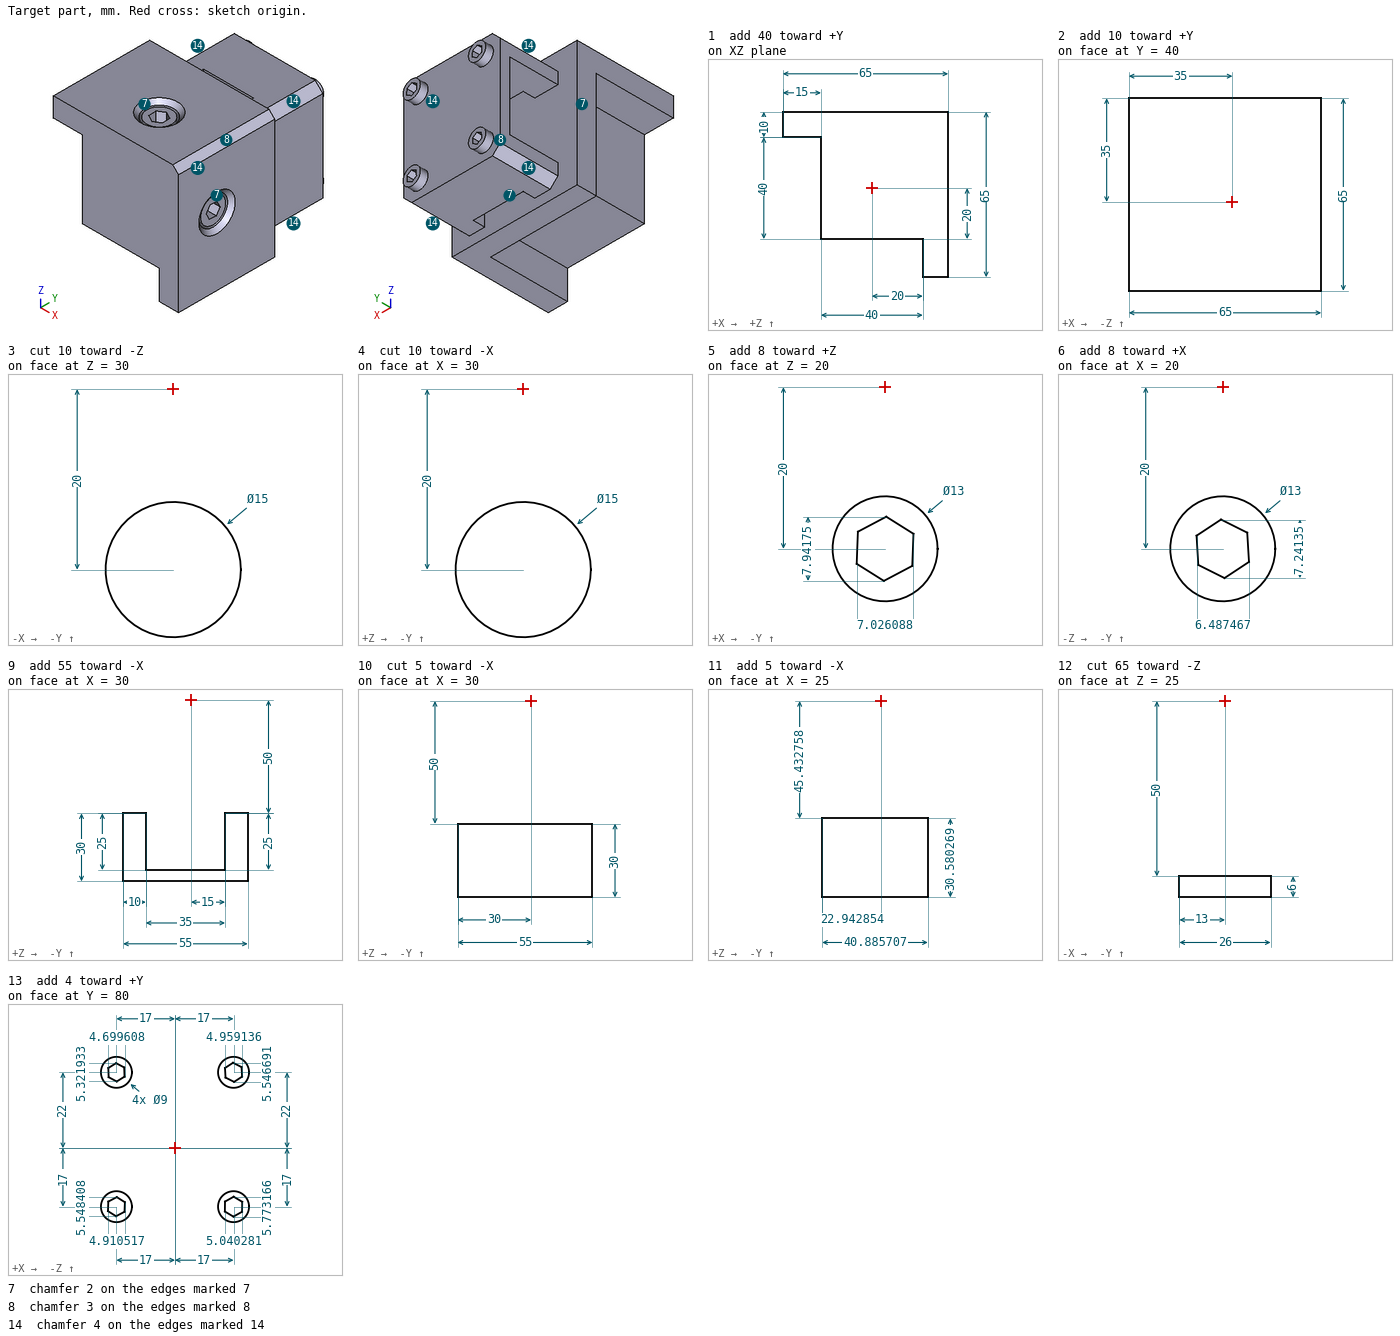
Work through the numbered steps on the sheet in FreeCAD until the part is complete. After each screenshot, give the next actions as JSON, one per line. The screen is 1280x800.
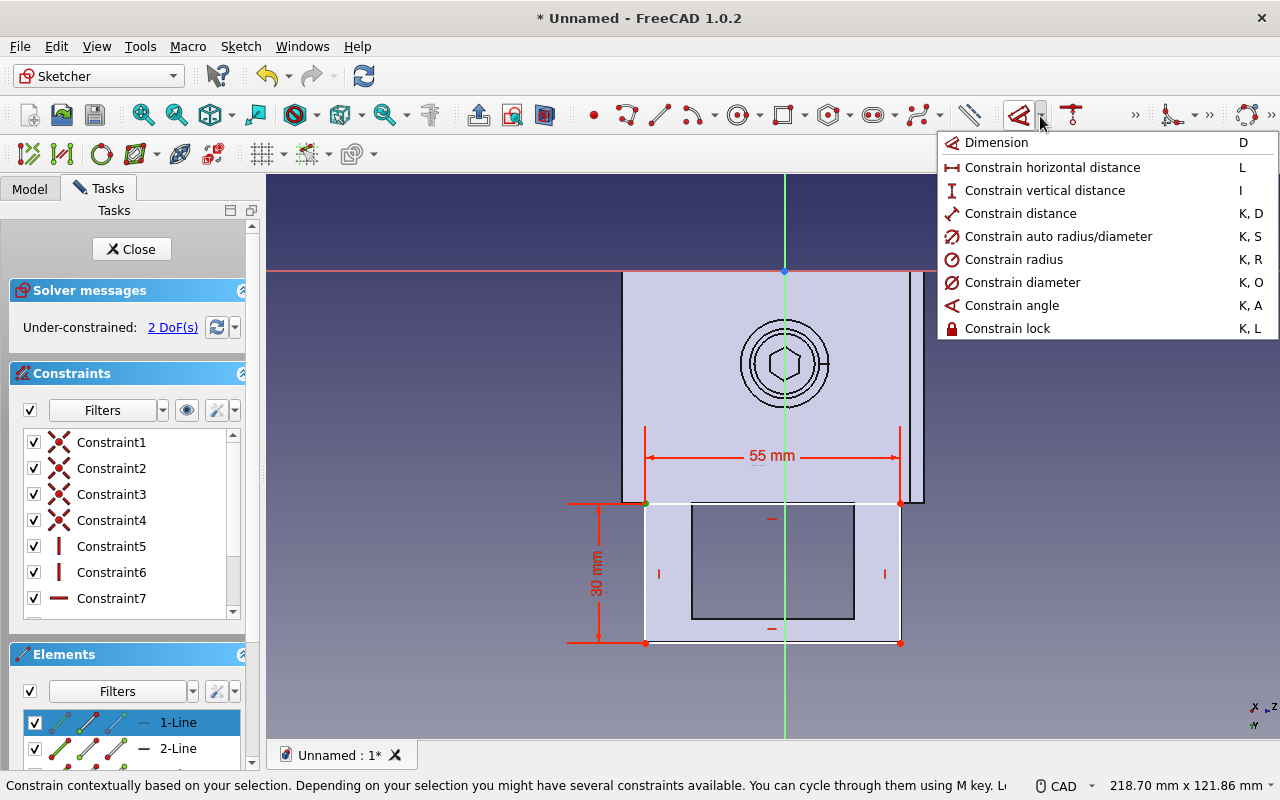
{"action": "left_click", "coordinate": [1108, 168]}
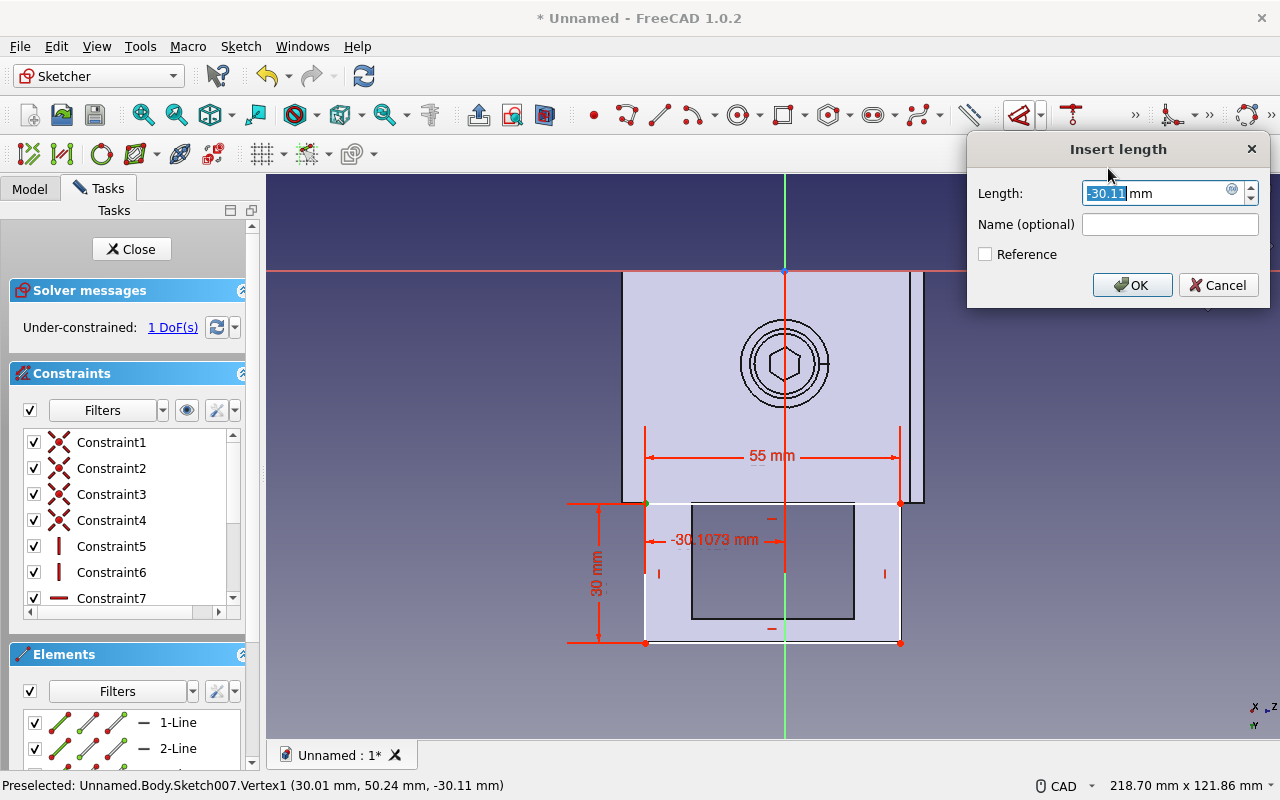
{"action": "type", "text": "-30"}
{"action": "key", "text": "Return"}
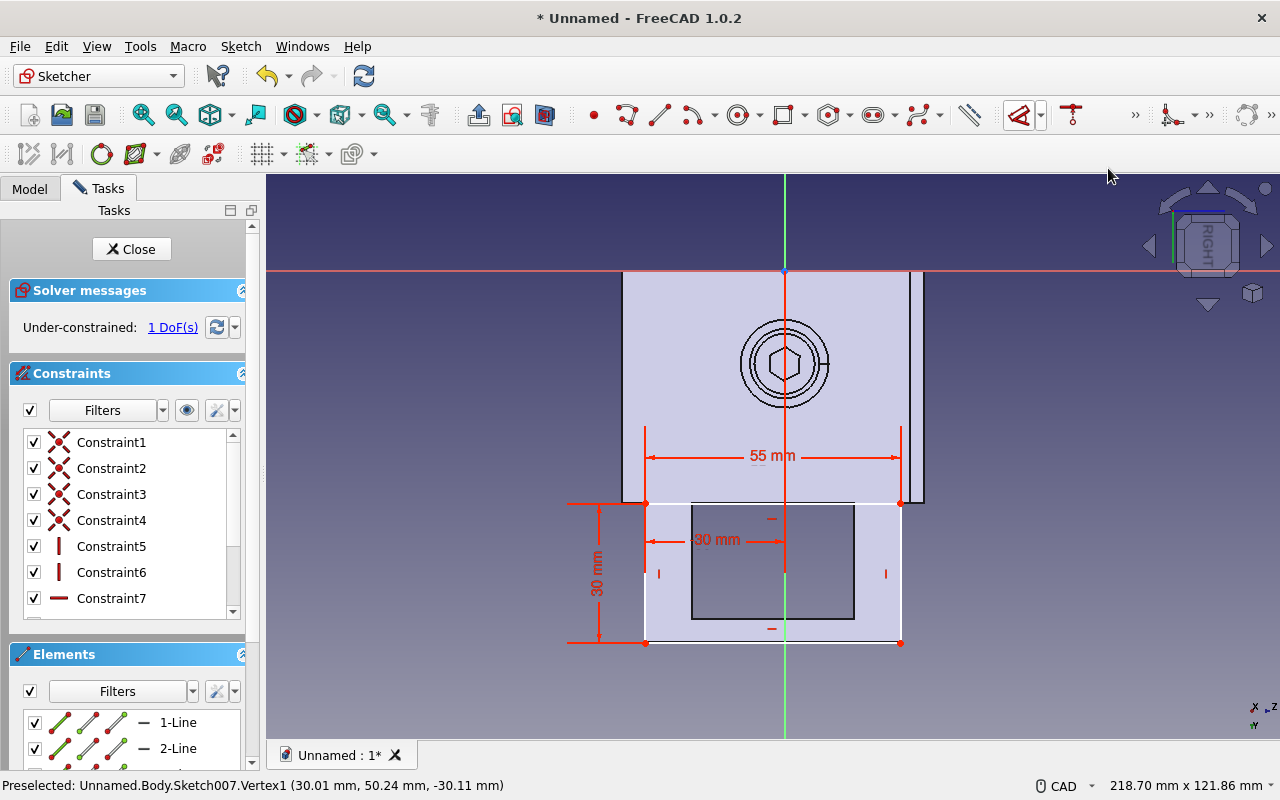
{"action": "left_click", "coordinate": [645, 504]}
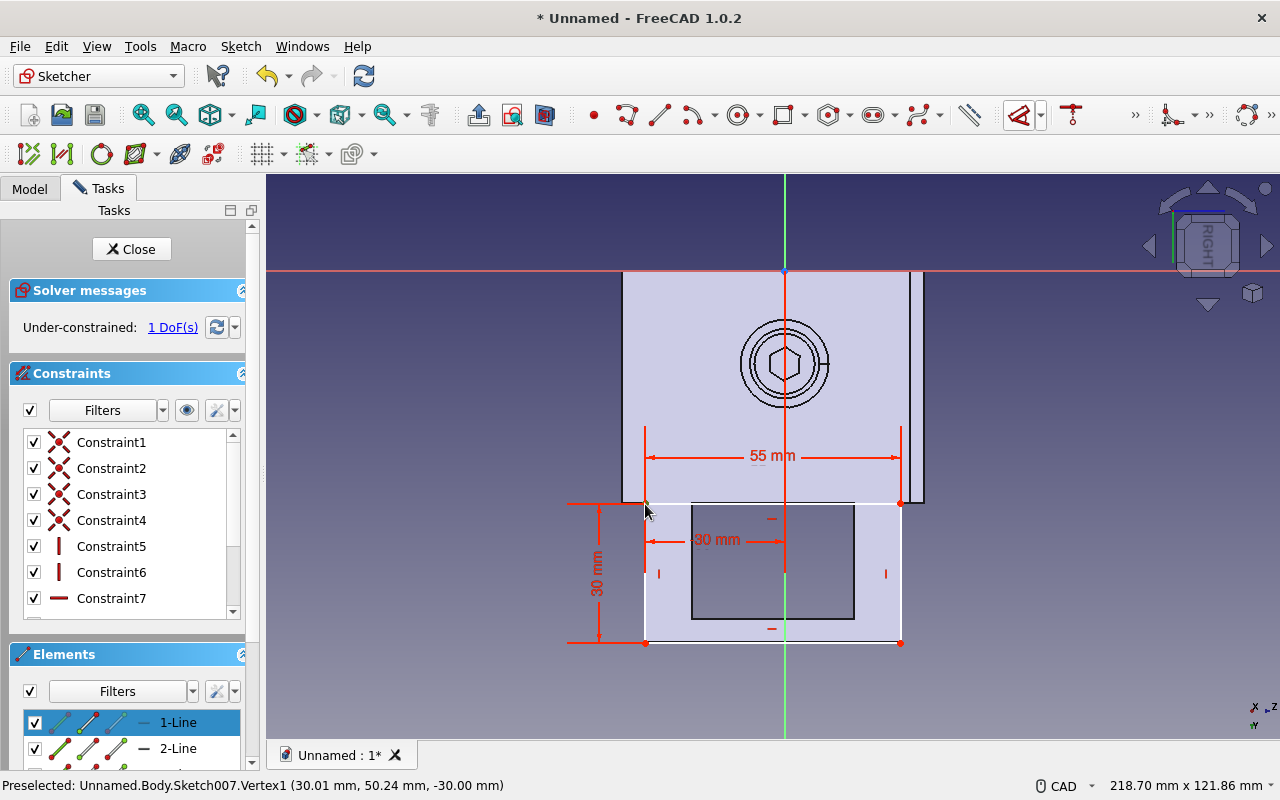
{"action": "left_click", "coordinate": [1040, 116]}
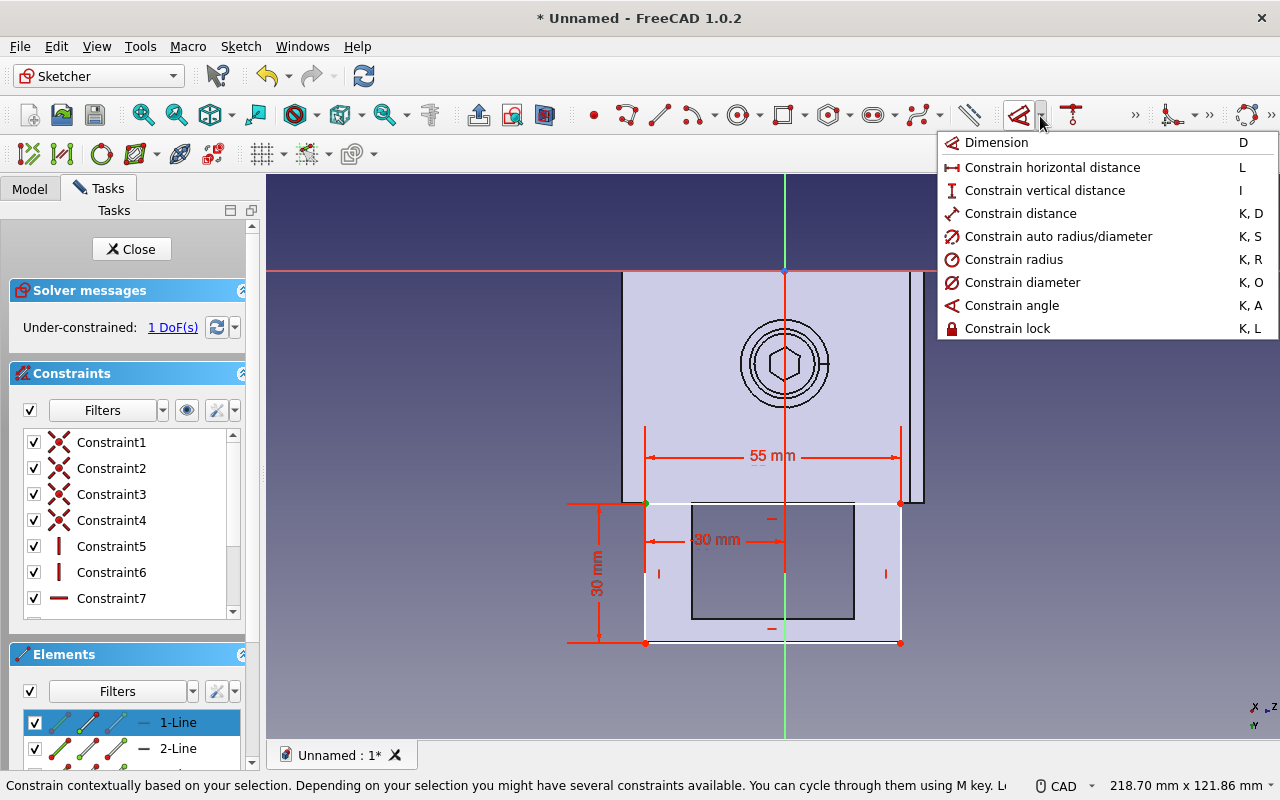
{"action": "left_click", "coordinate": [1108, 190]}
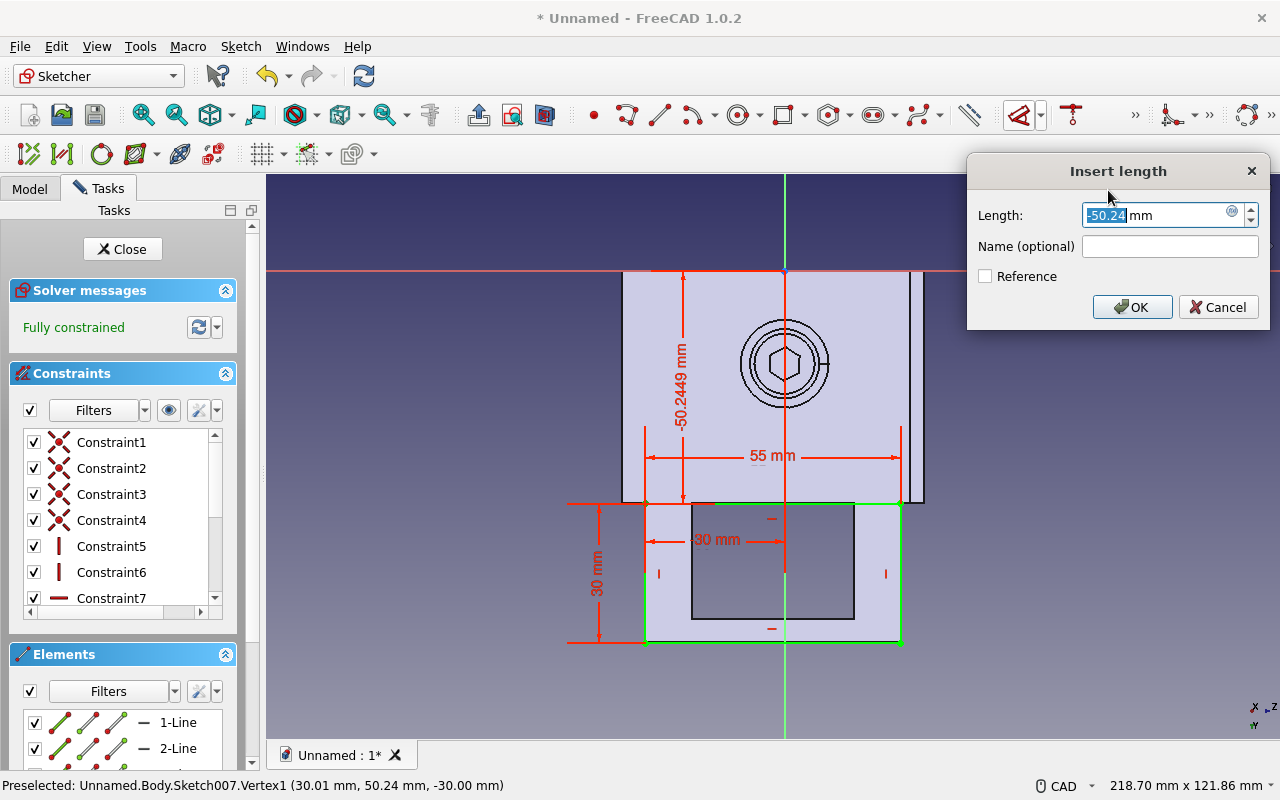
{"action": "type", "text": "-50"}
{"action": "key", "text": "Return"}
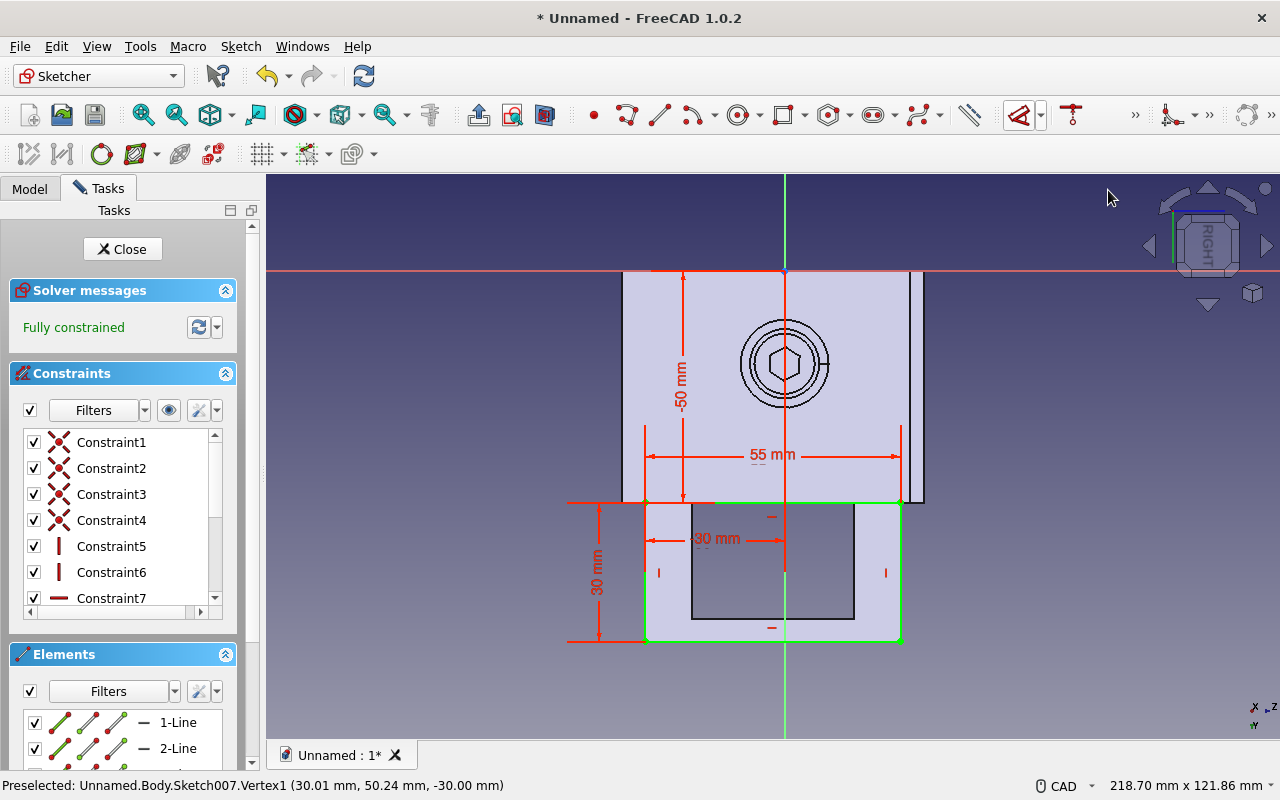
{"action": "left_click", "coordinate": [123, 249]}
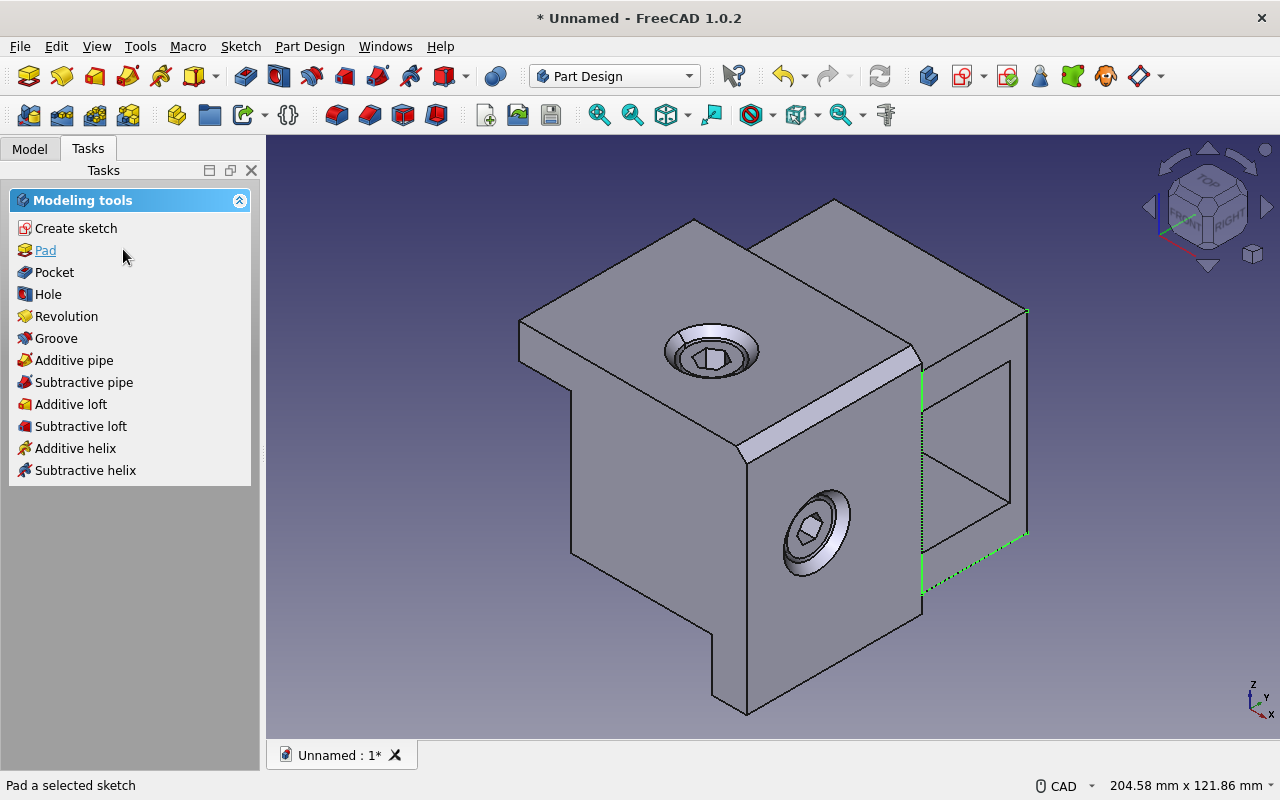
{"action": "left_click", "coordinate": [246, 76]}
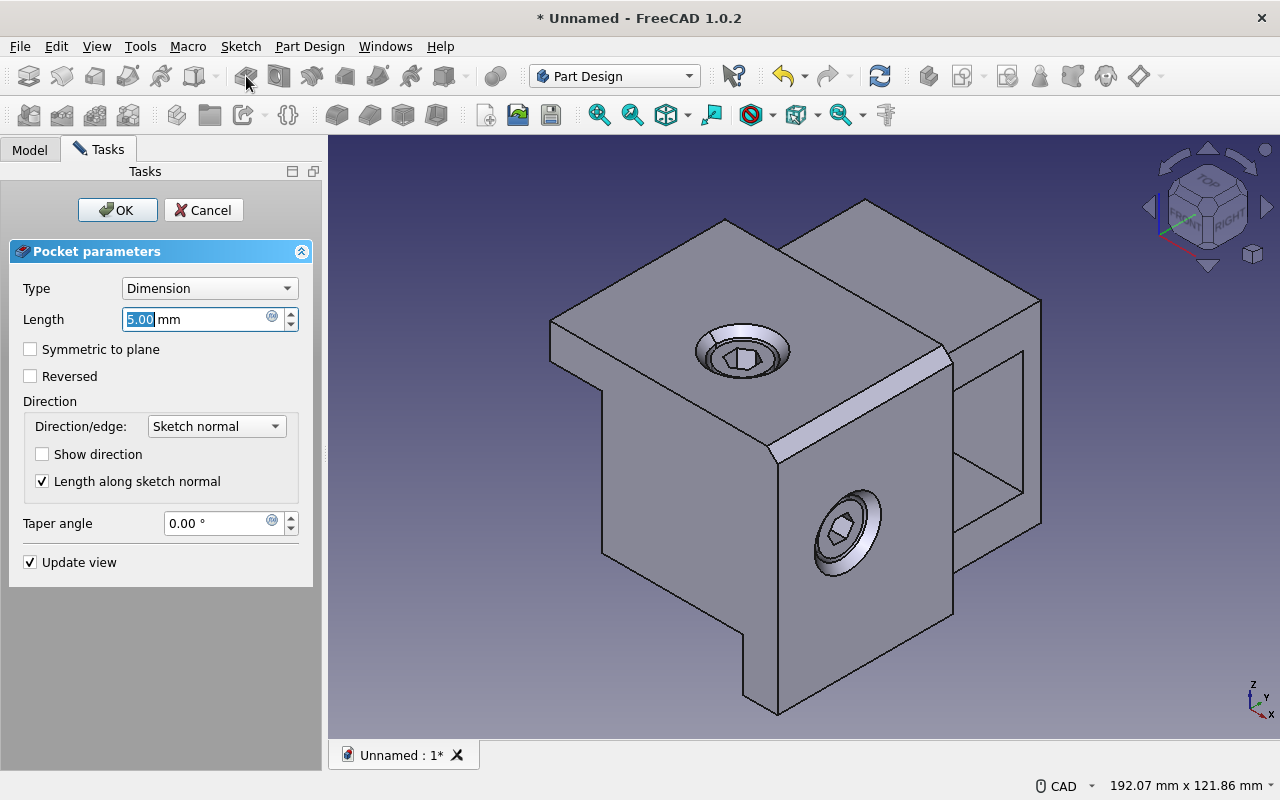
{"action": "type", "text": "5"}
{"action": "key", "text": "Tab"}